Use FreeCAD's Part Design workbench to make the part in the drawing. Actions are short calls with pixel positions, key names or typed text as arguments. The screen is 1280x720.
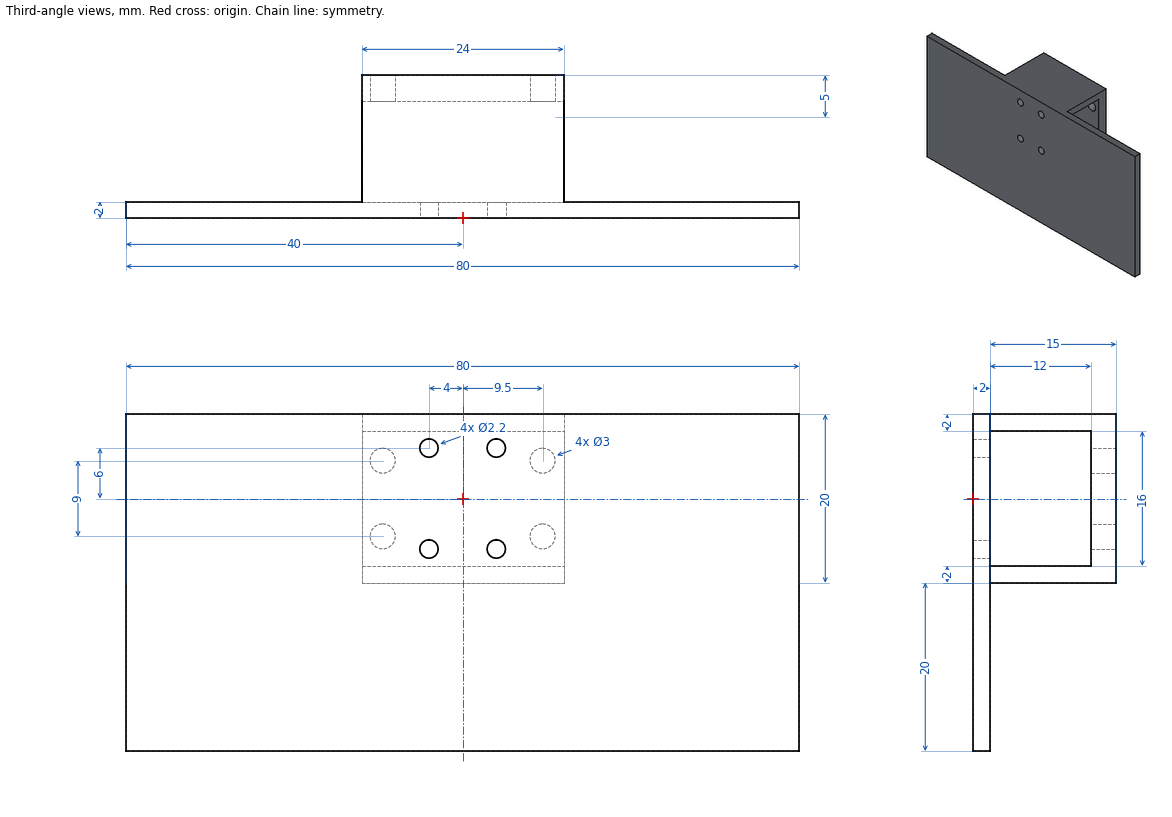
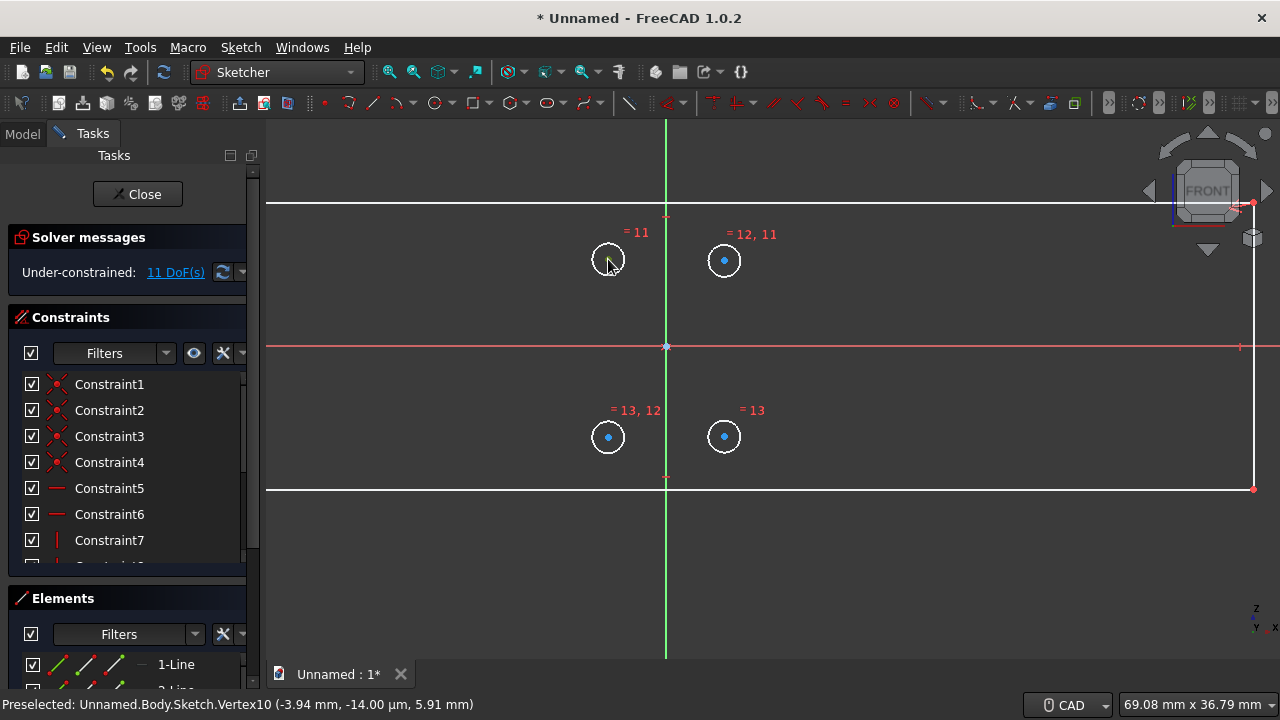
click(724, 261)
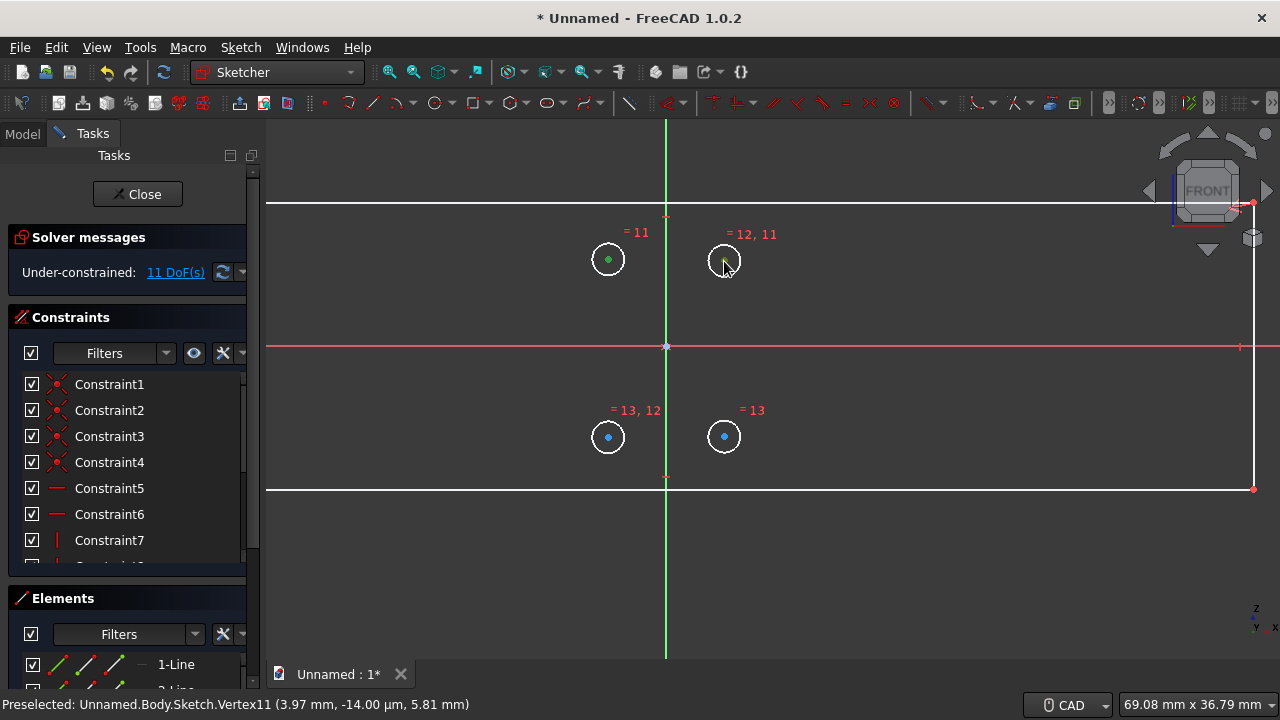
click(666, 596)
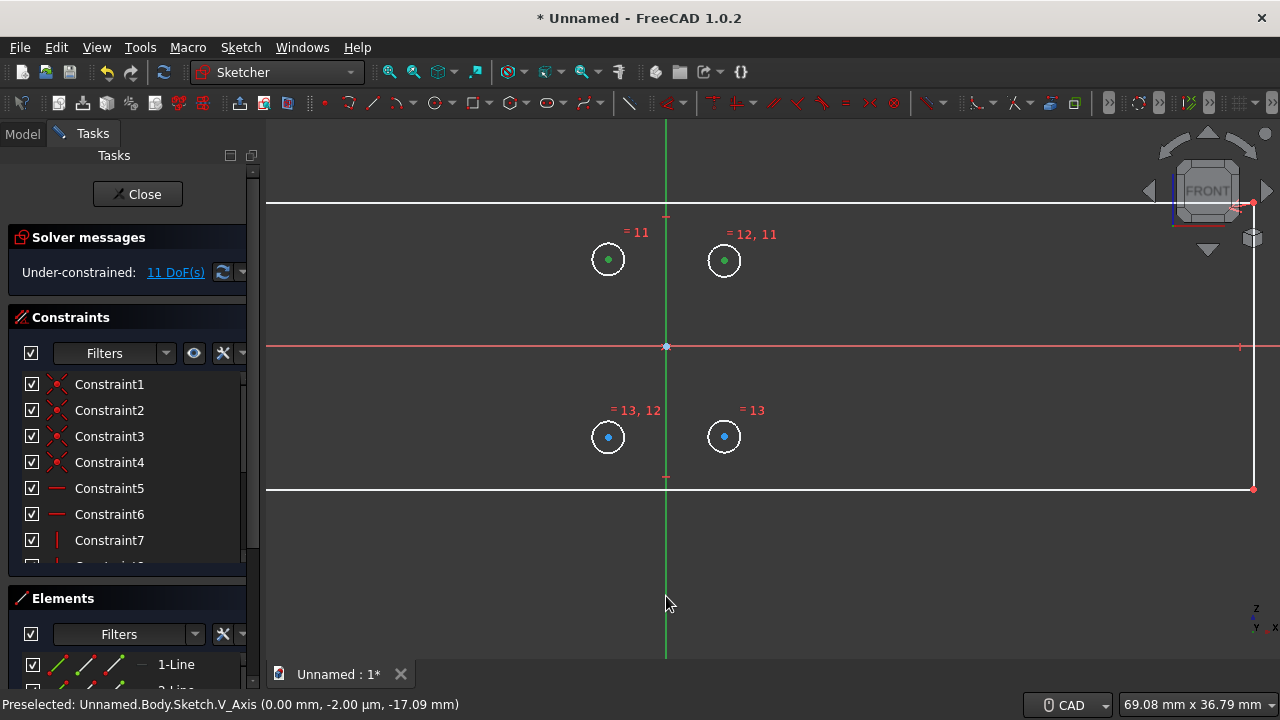
click(870, 104)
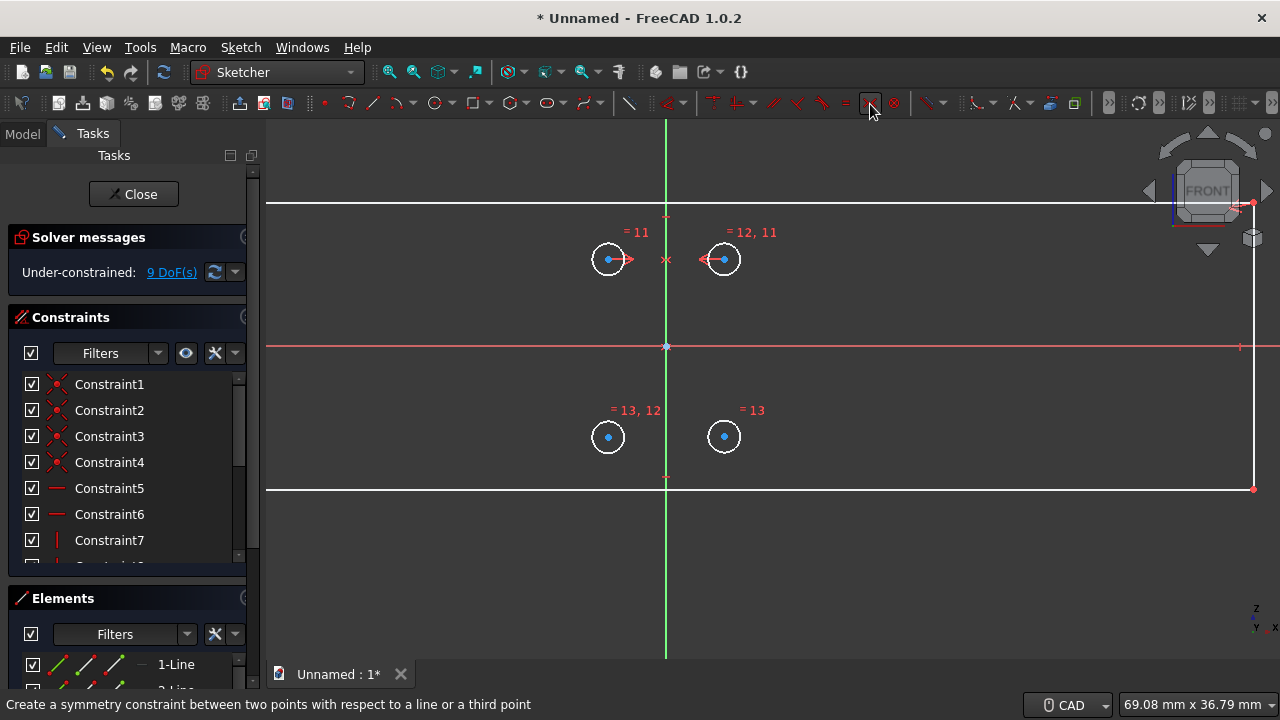
click(608, 259)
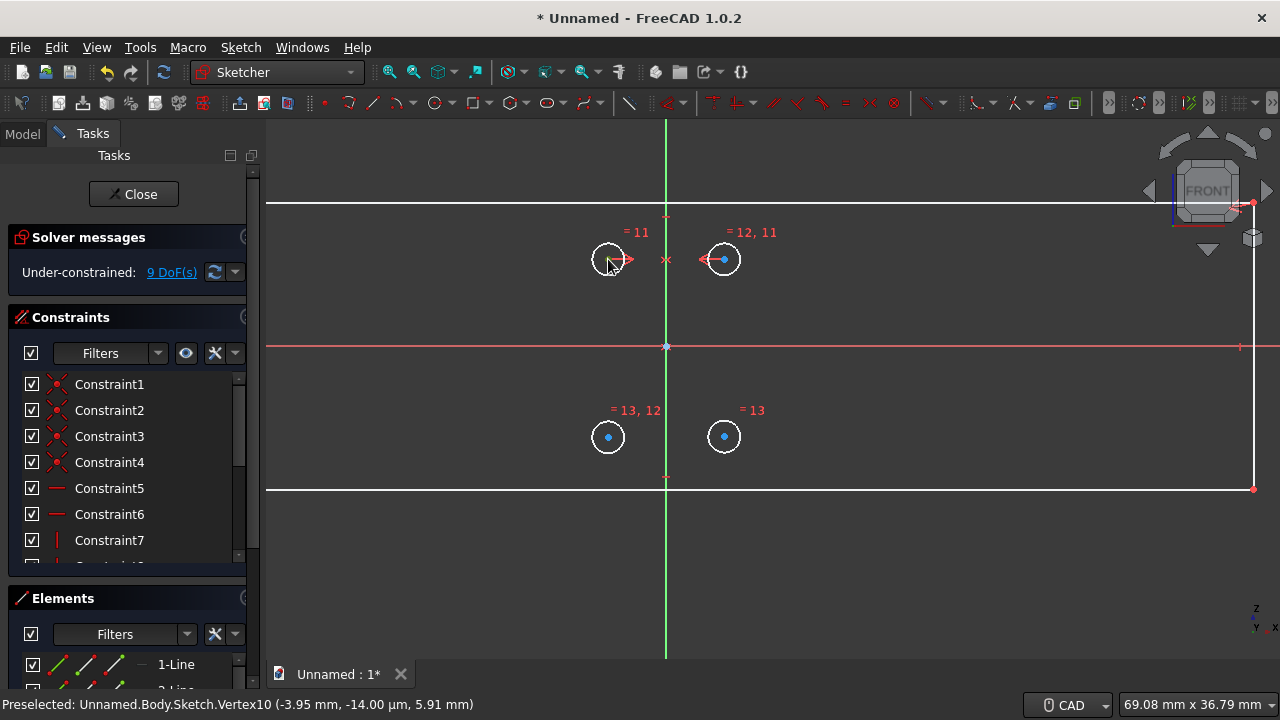
click(608, 437)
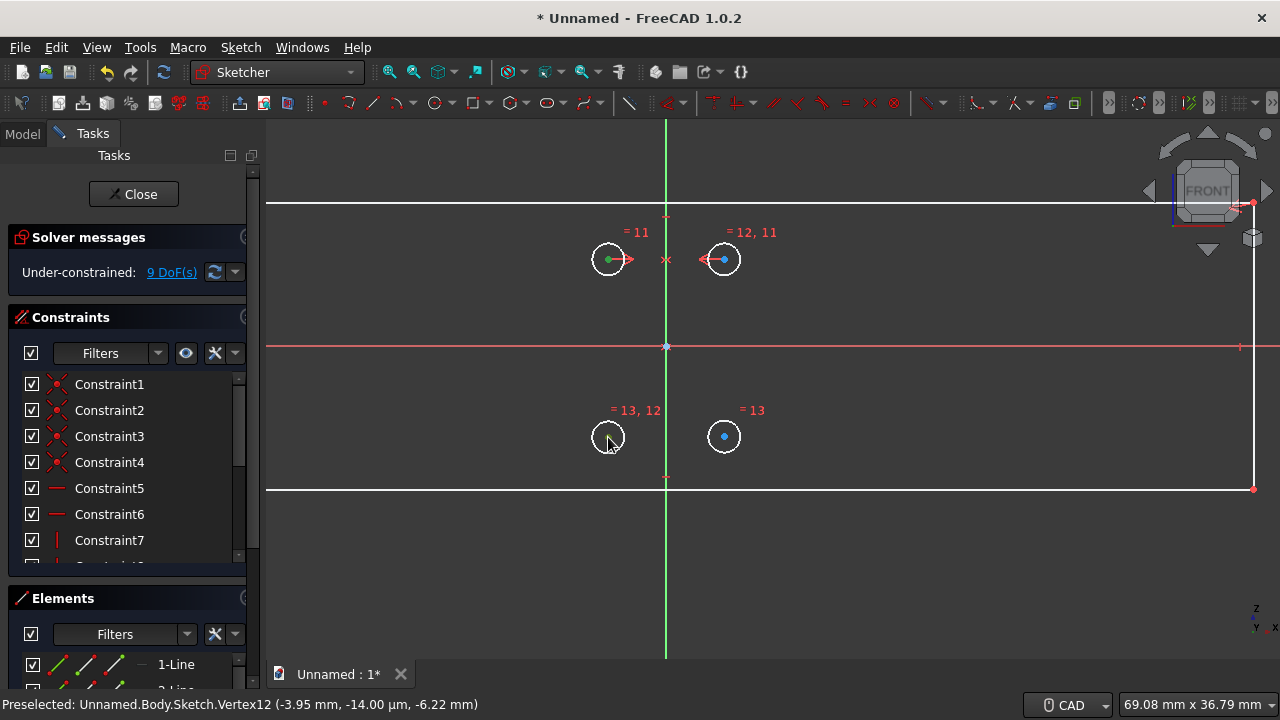
click(353, 346)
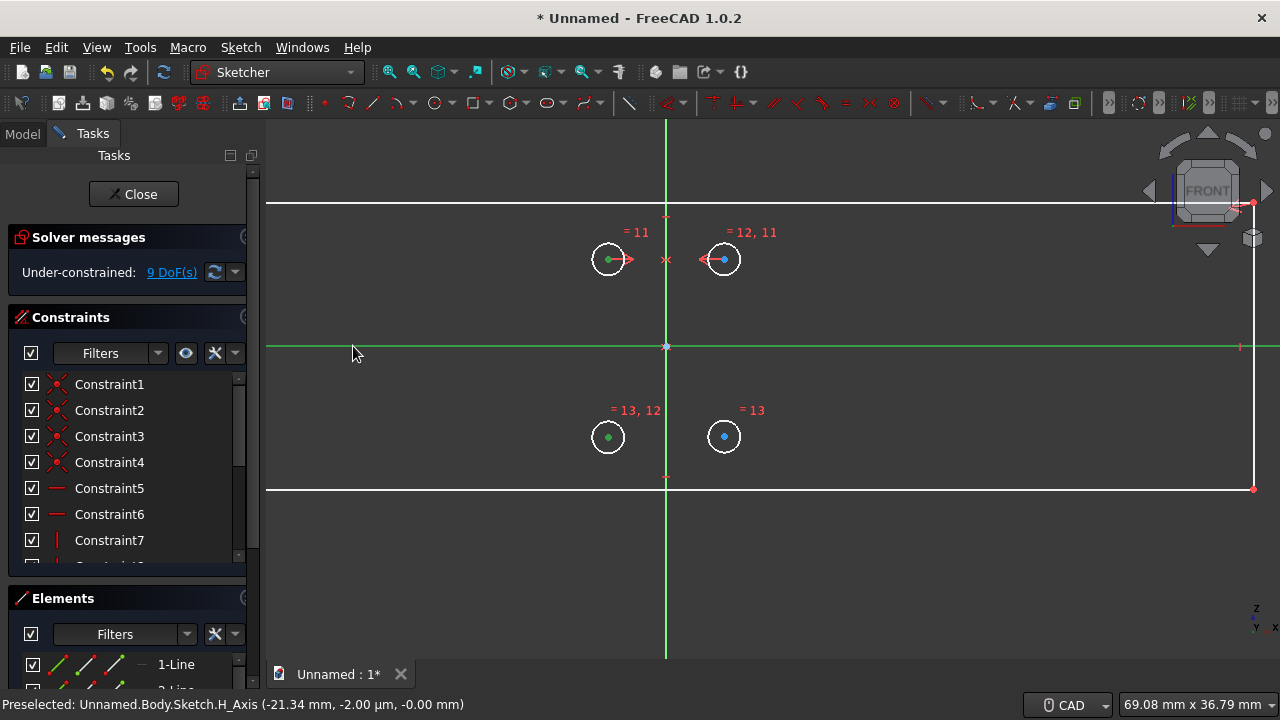
click(870, 104)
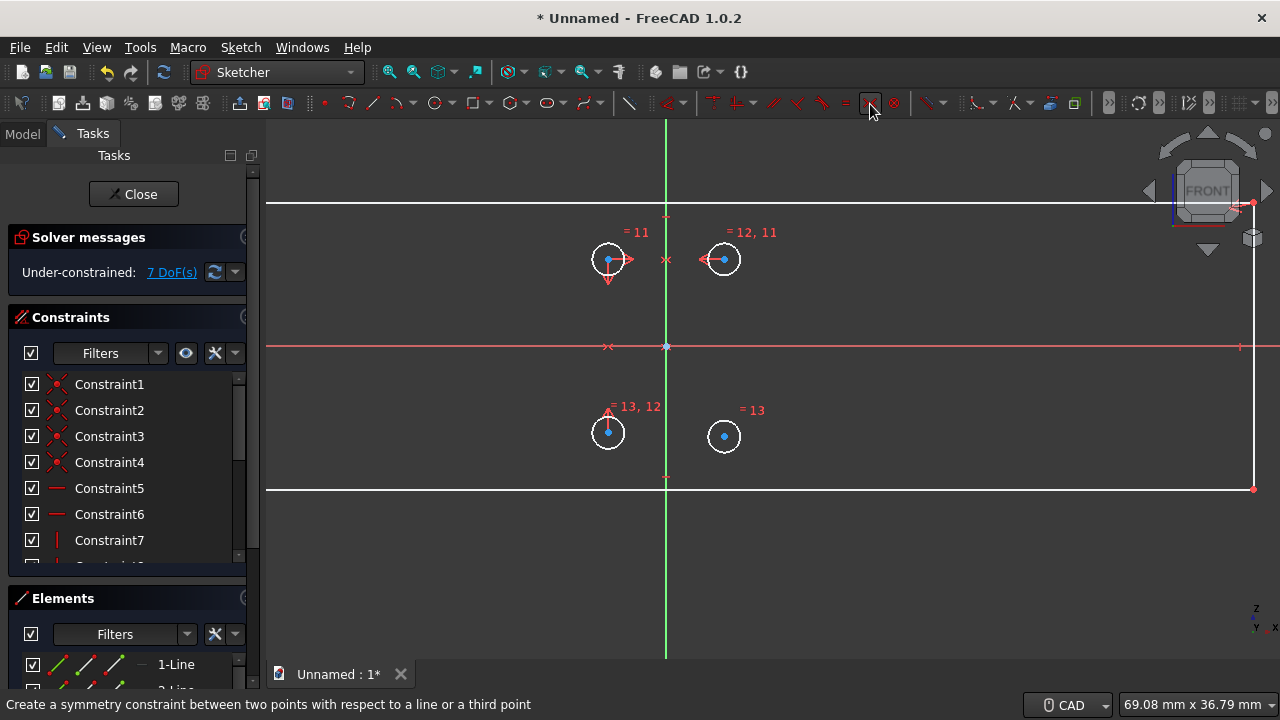
click(724, 259)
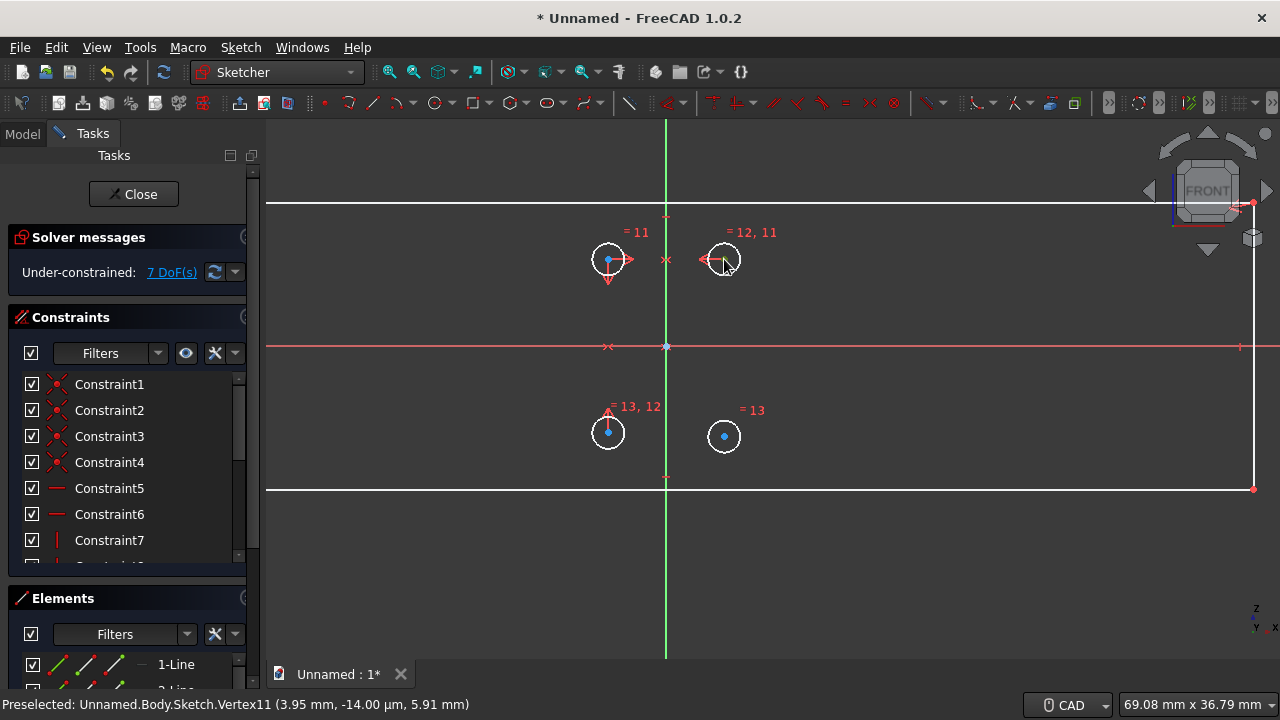
click(724, 437)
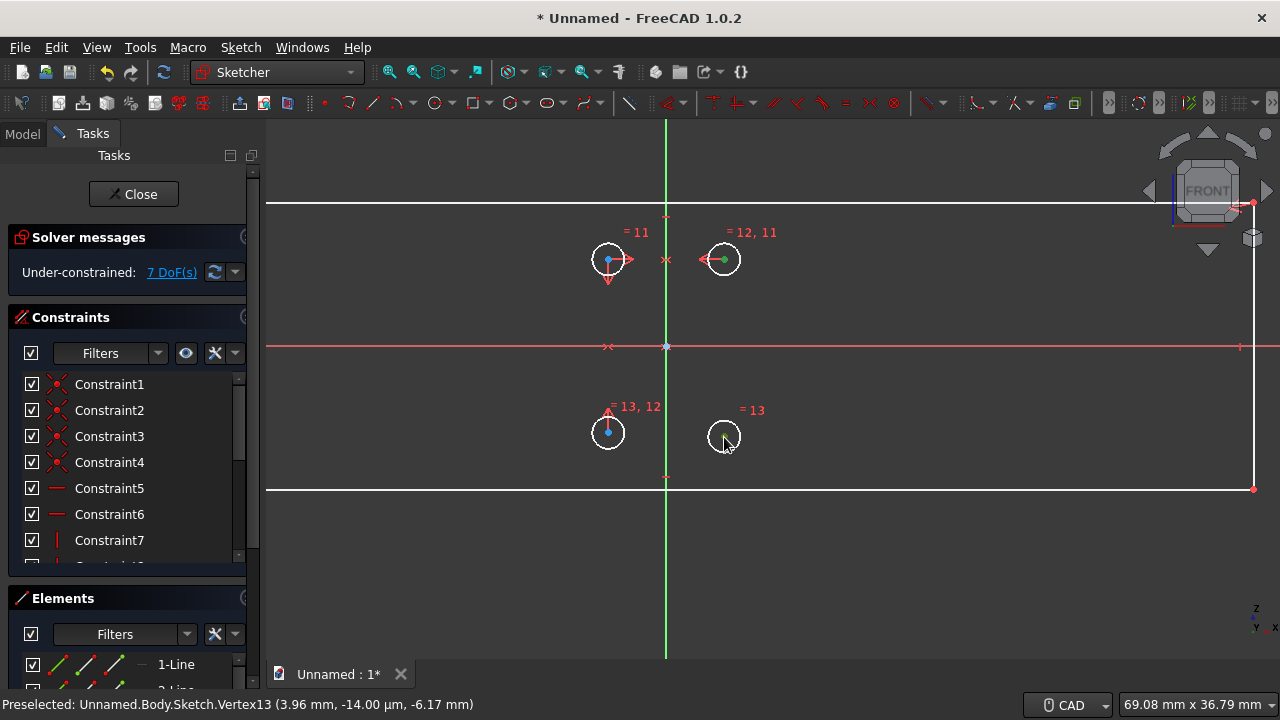
click(353, 346)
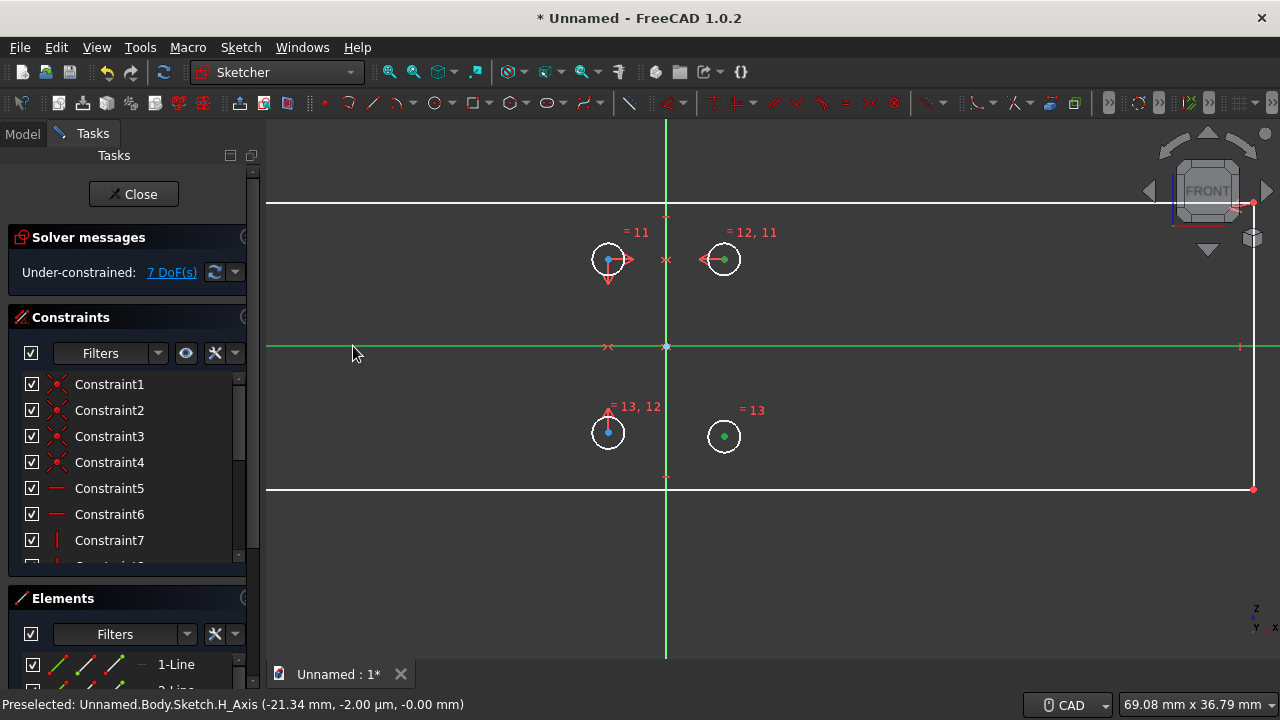
click(870, 104)